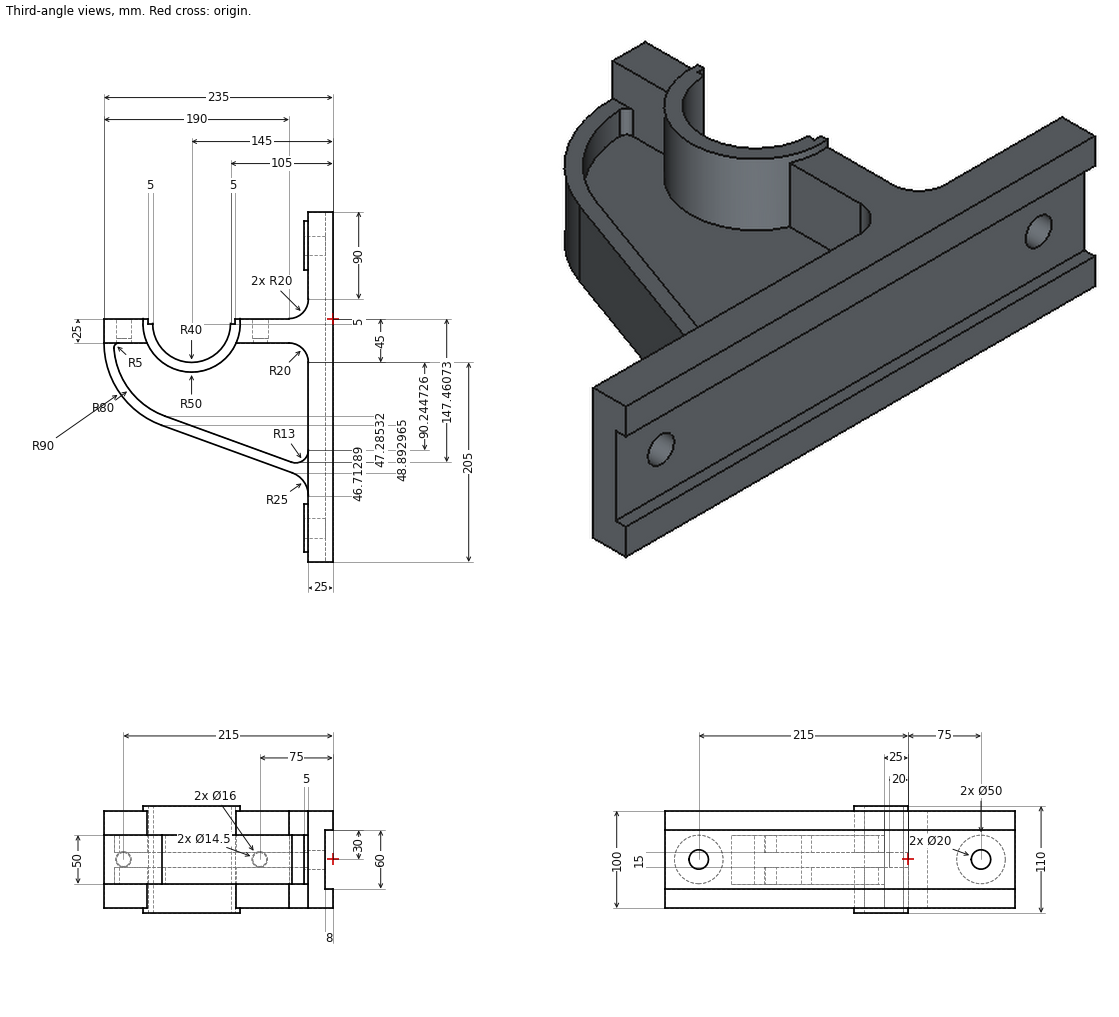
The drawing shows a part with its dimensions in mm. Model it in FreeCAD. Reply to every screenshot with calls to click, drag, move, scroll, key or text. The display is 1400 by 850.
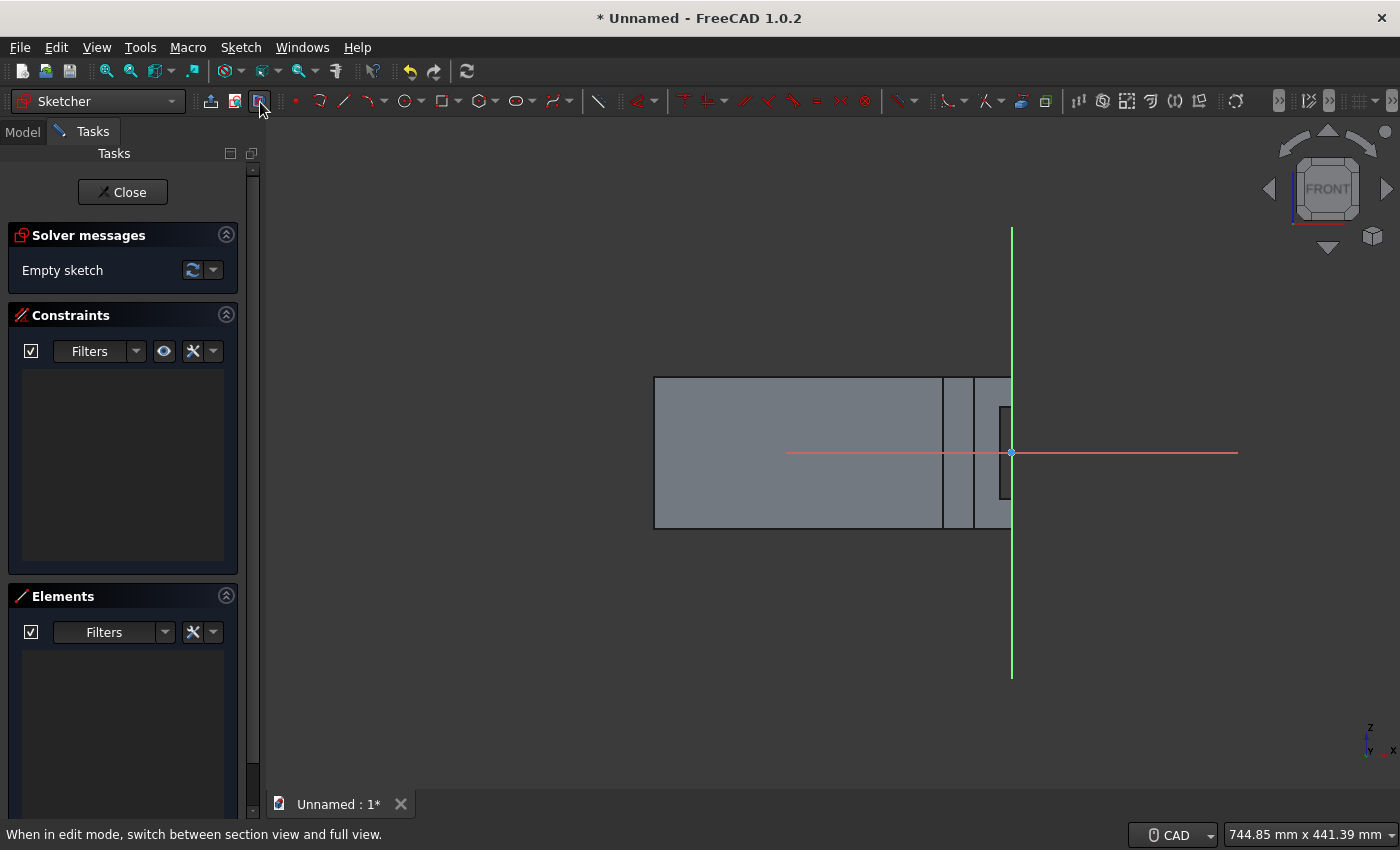
scroll(938, 453, up, 3)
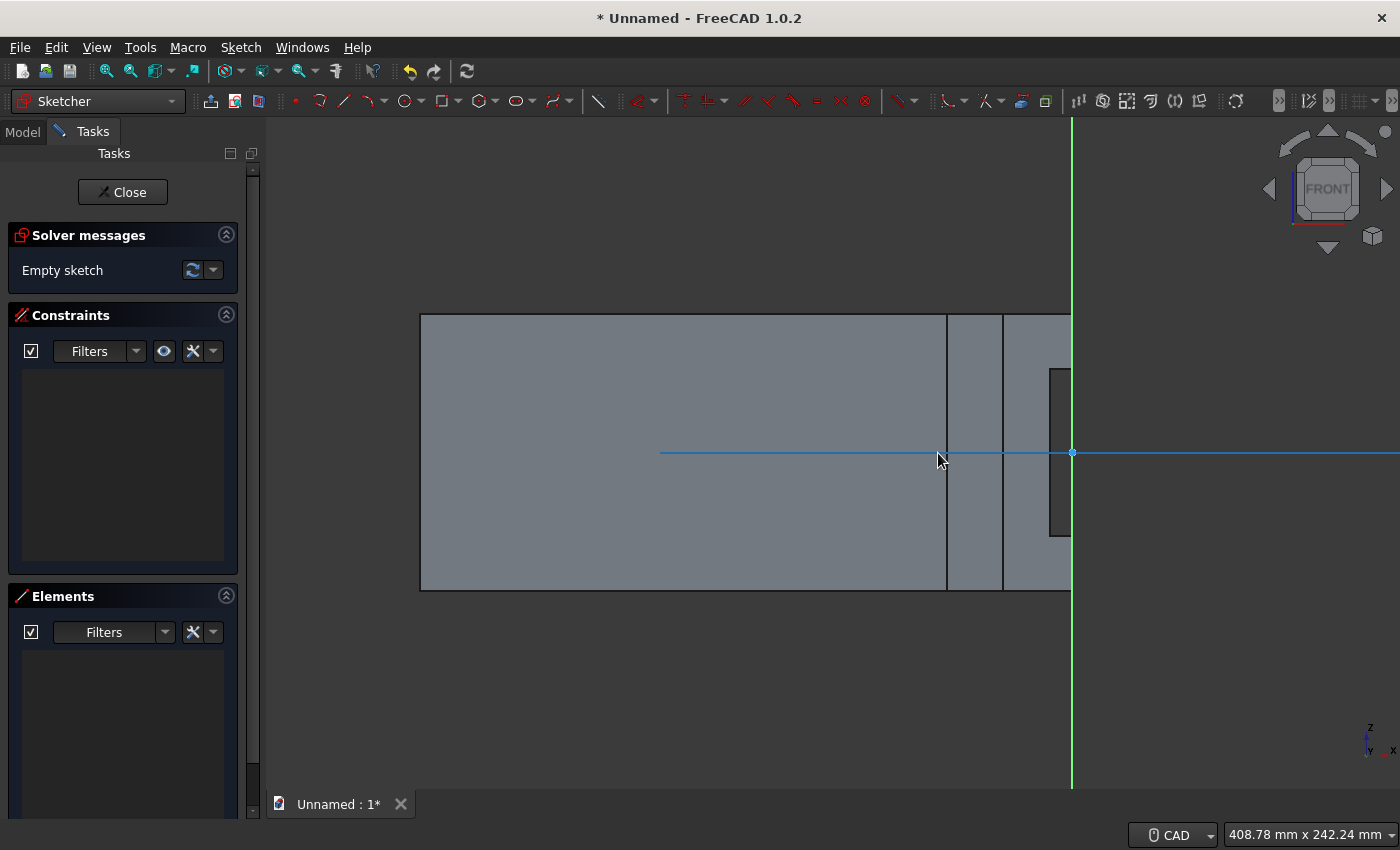
click(406, 102)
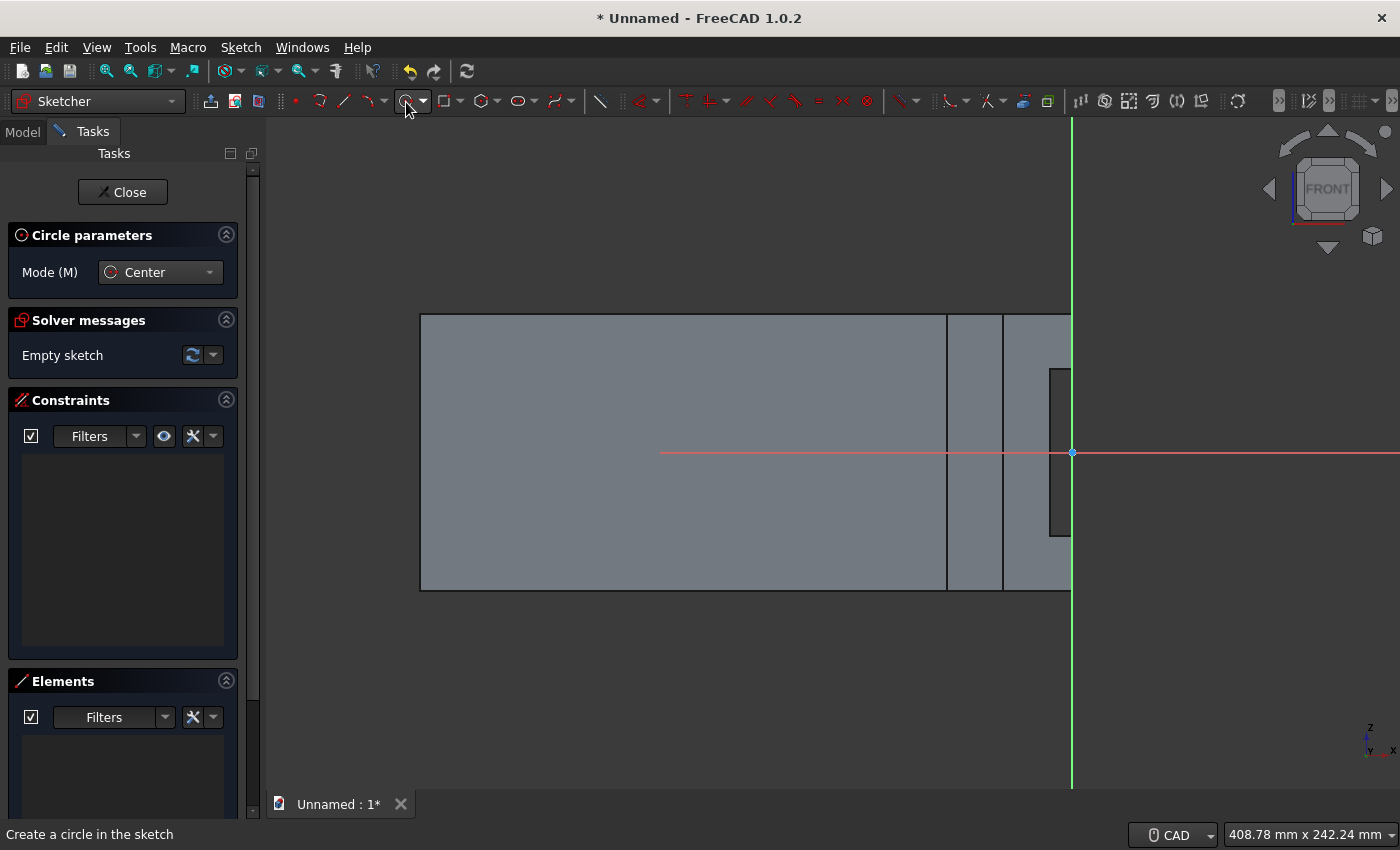
click(864, 453)
move(878, 438)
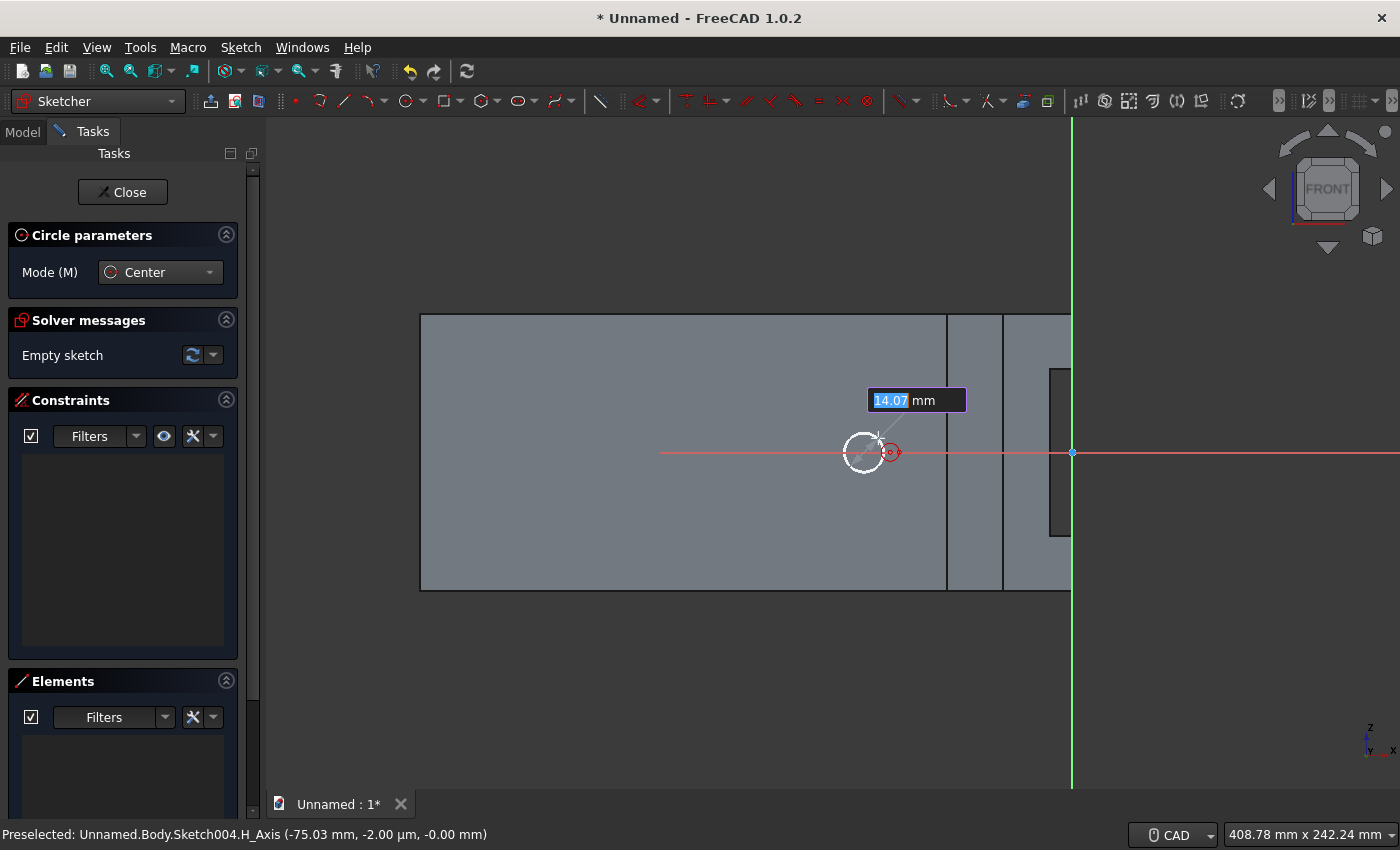
text(14.5)
key(Return)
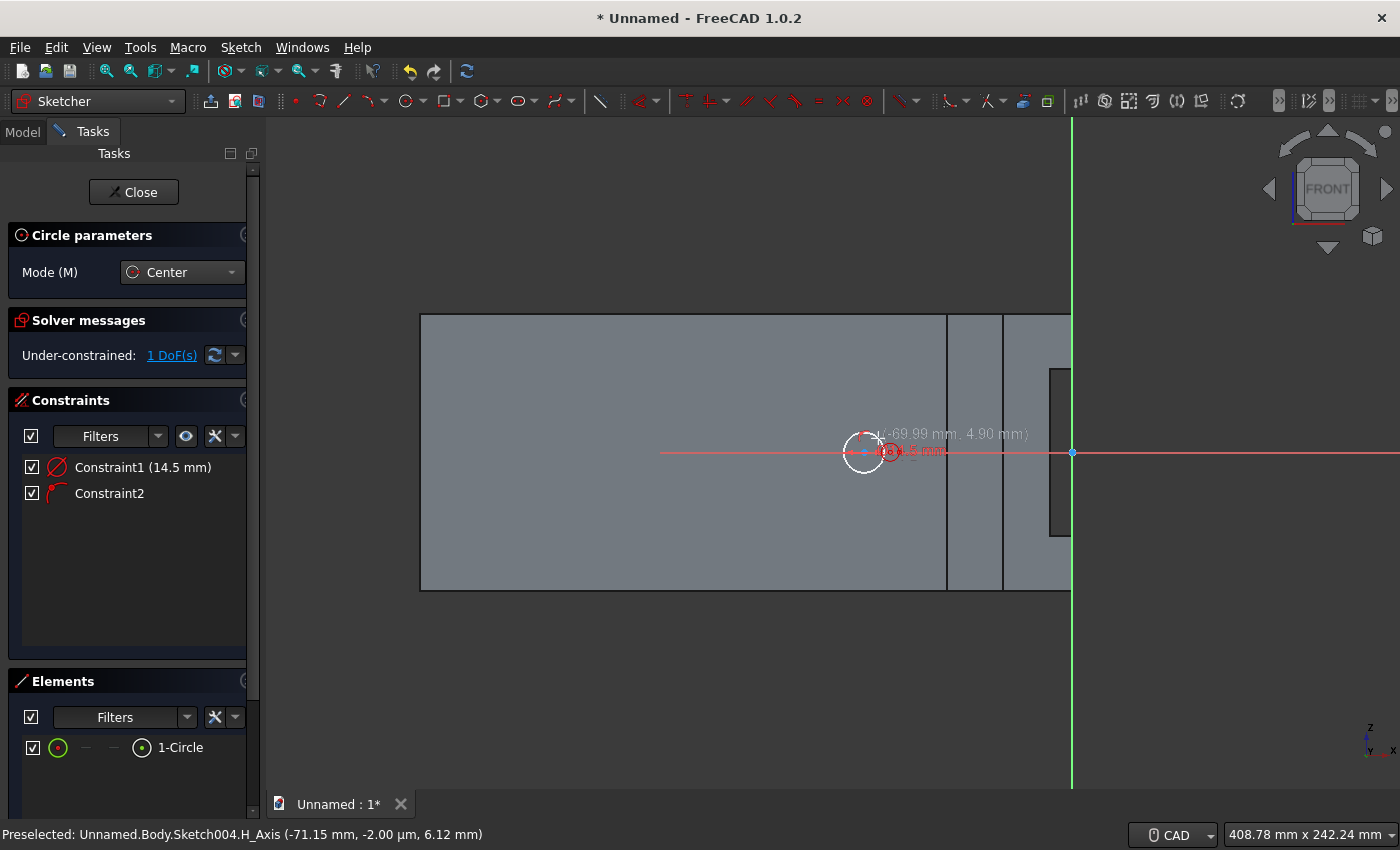
click(476, 453)
move(490, 438)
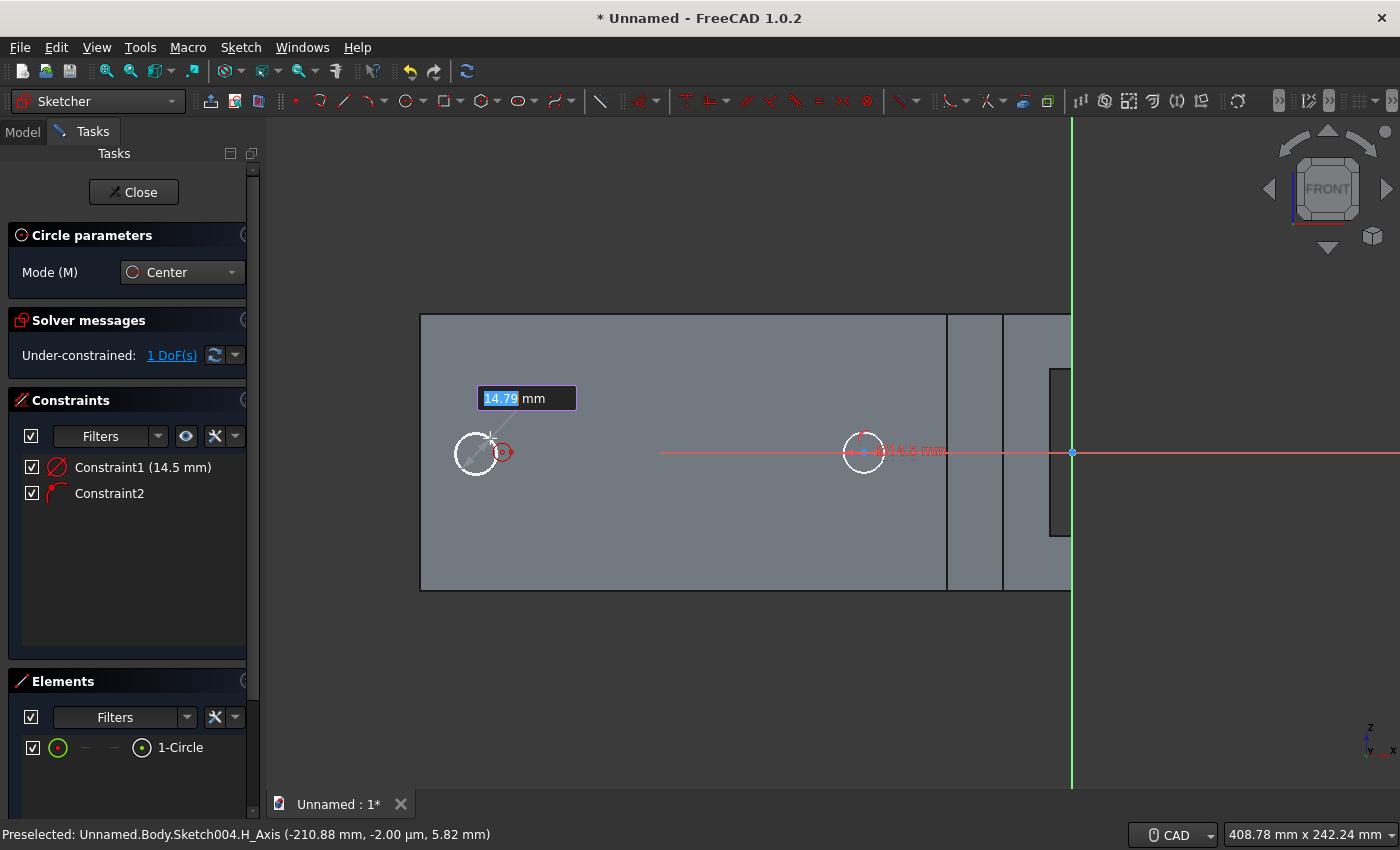
text(14.5)
key(Return)
key(Escape)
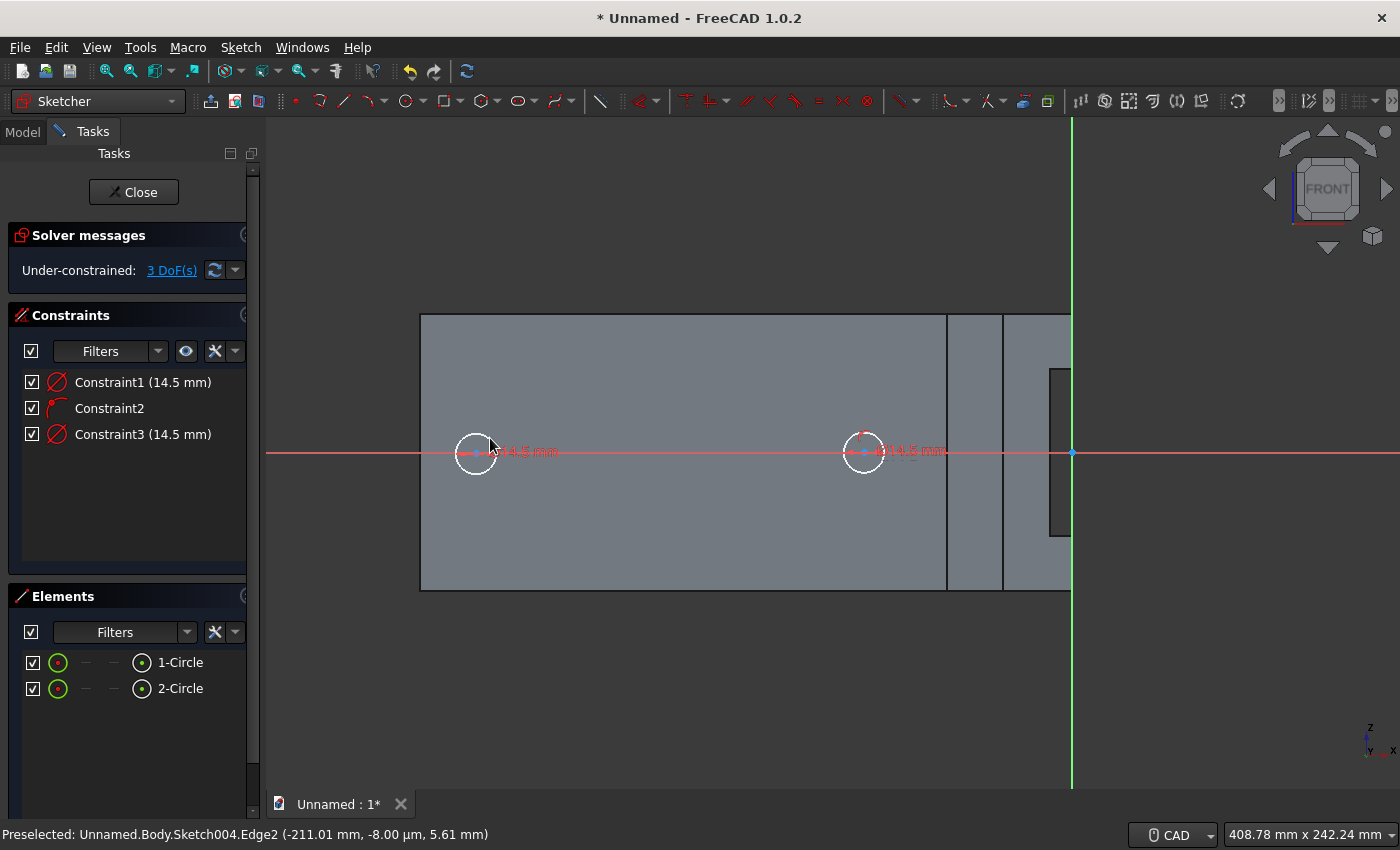
click(476, 454)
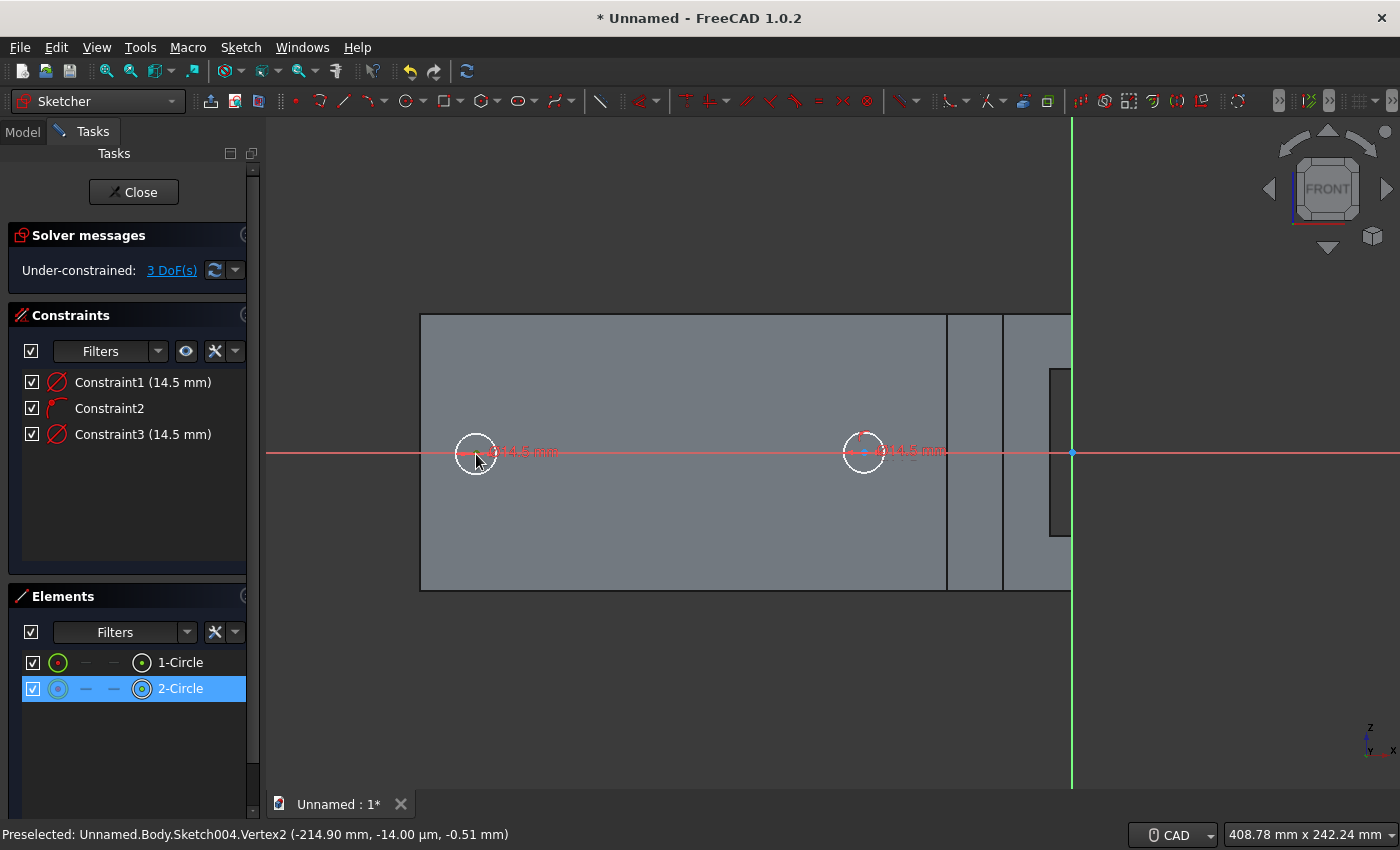
click(361, 453)